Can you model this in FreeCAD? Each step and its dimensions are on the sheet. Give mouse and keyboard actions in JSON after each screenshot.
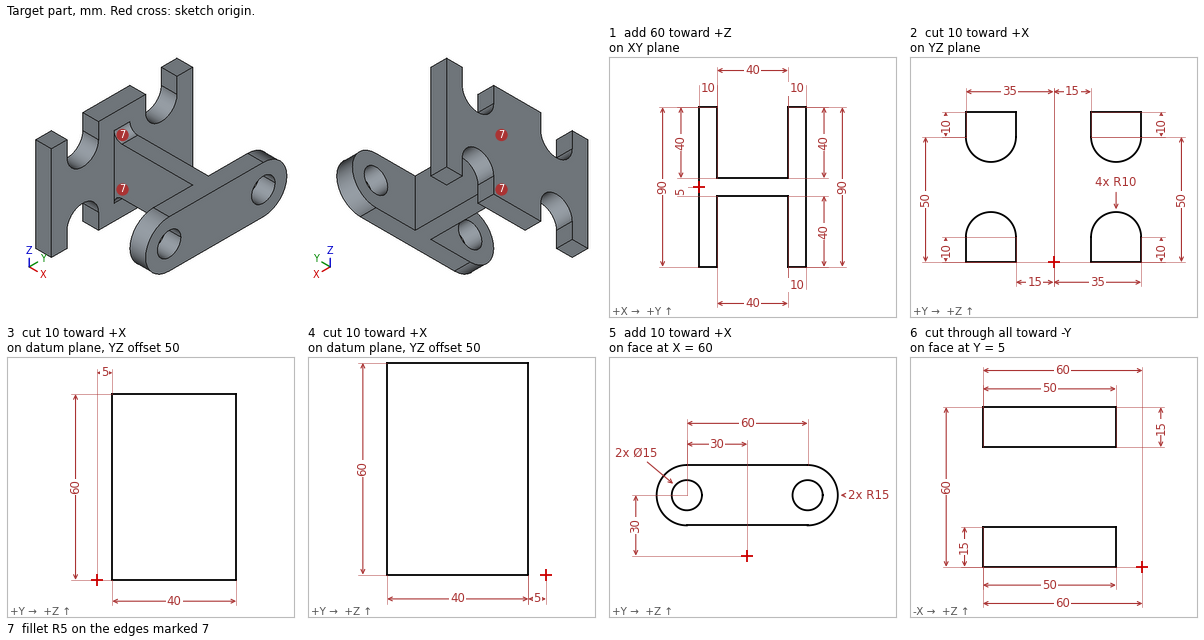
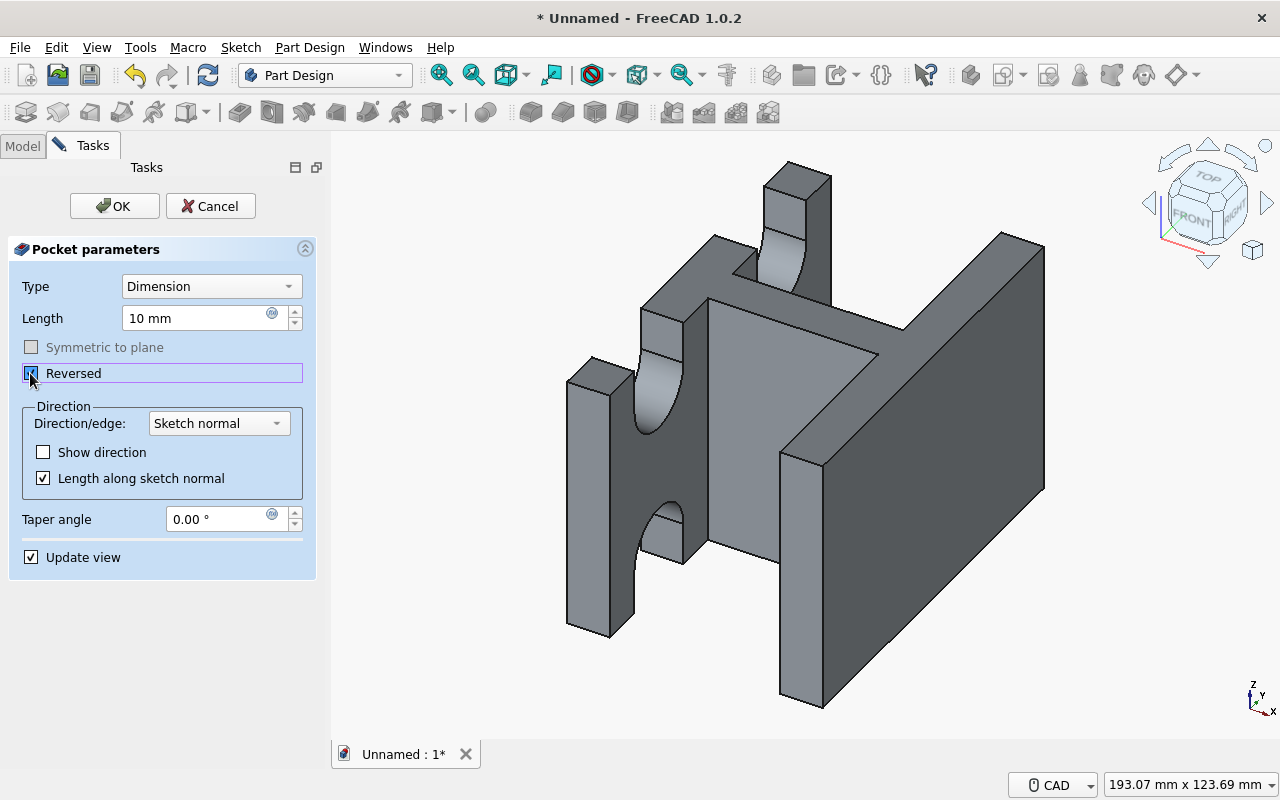
{"action": "left_click", "coordinate": [115, 206]}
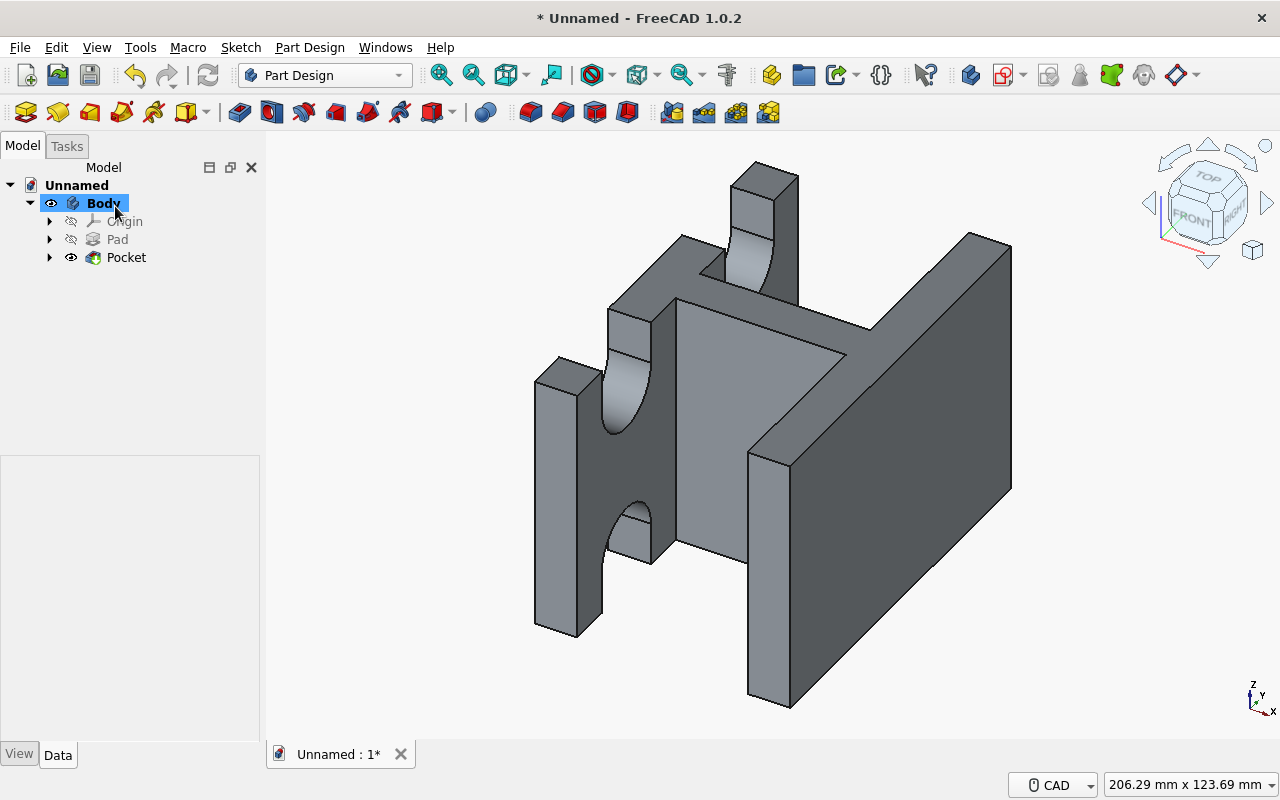
{"action": "left_click", "coordinate": [50, 221]}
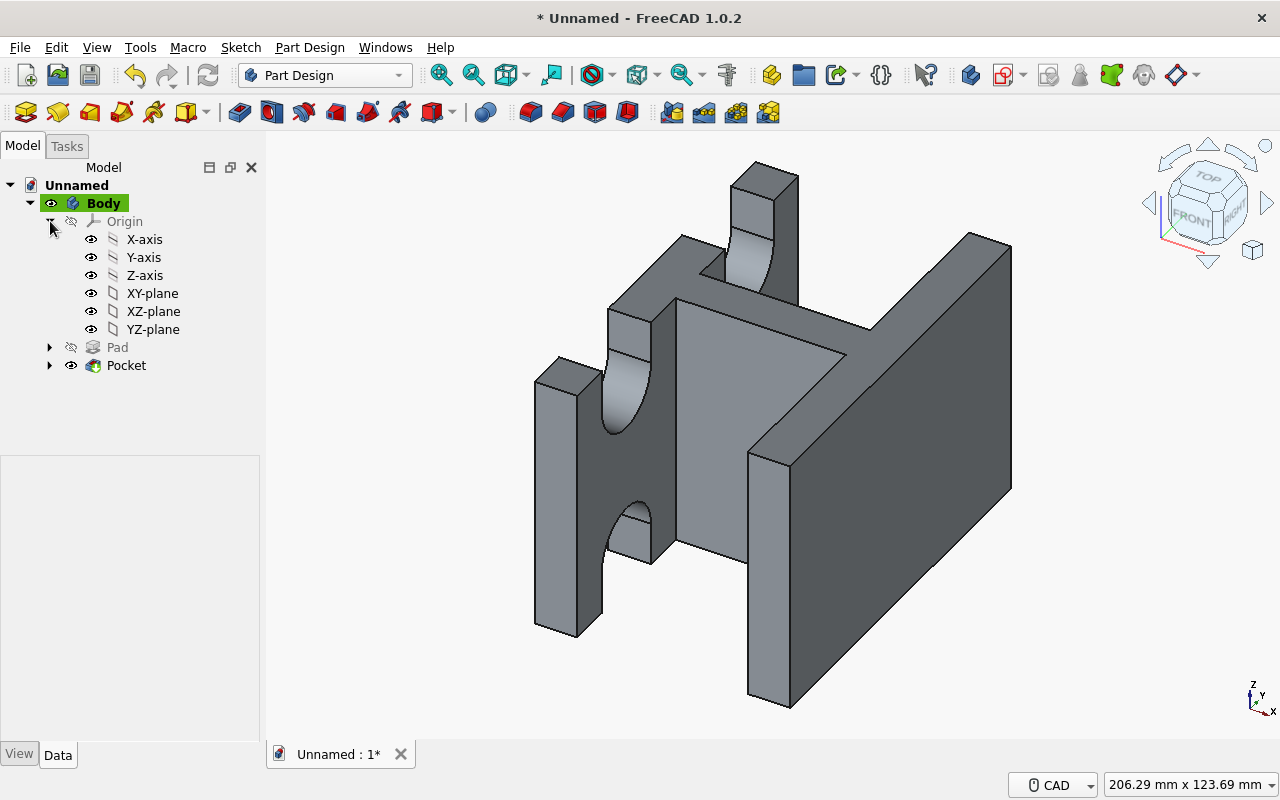
{"action": "left_click", "coordinate": [136, 329]}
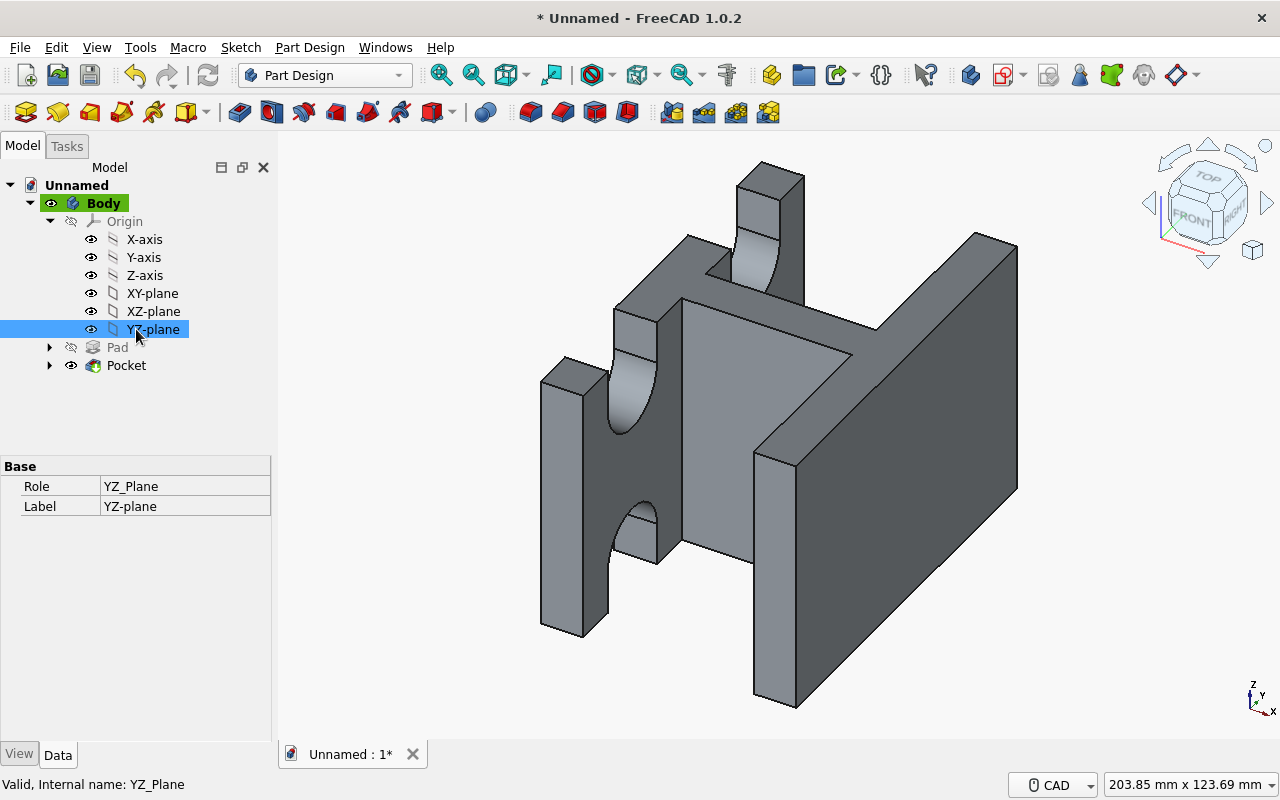
{"action": "left_click", "coordinate": [1176, 76]}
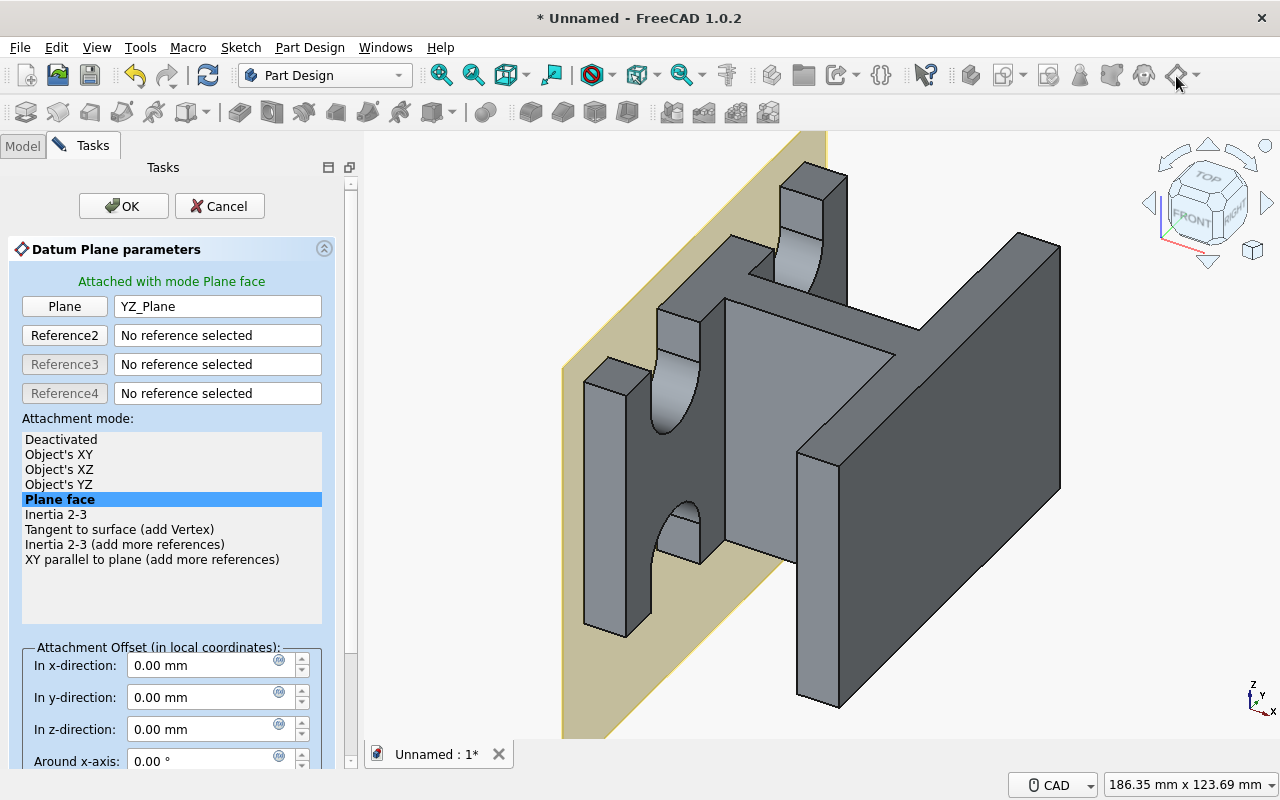
{"action": "triple_click", "coordinate": [210, 729]}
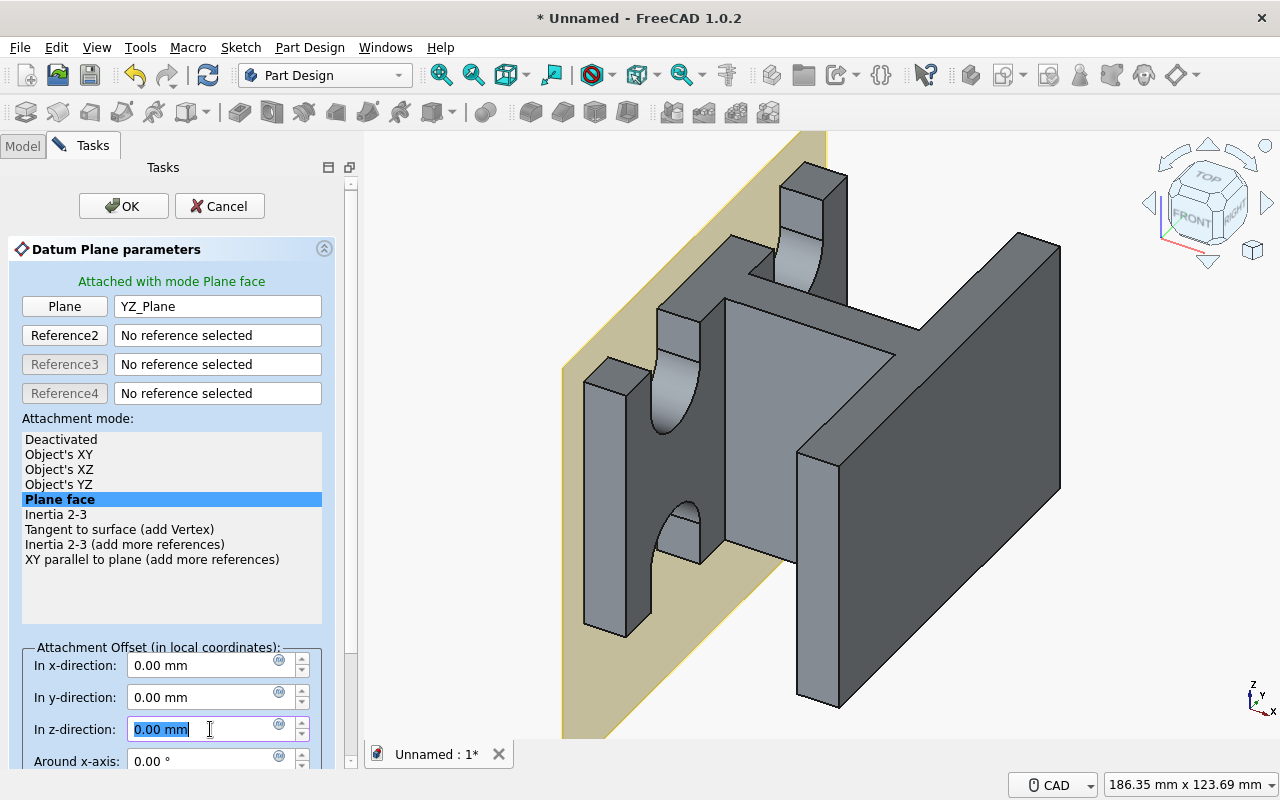
{"action": "type", "text": "50"}
{"action": "key", "text": "Tab"}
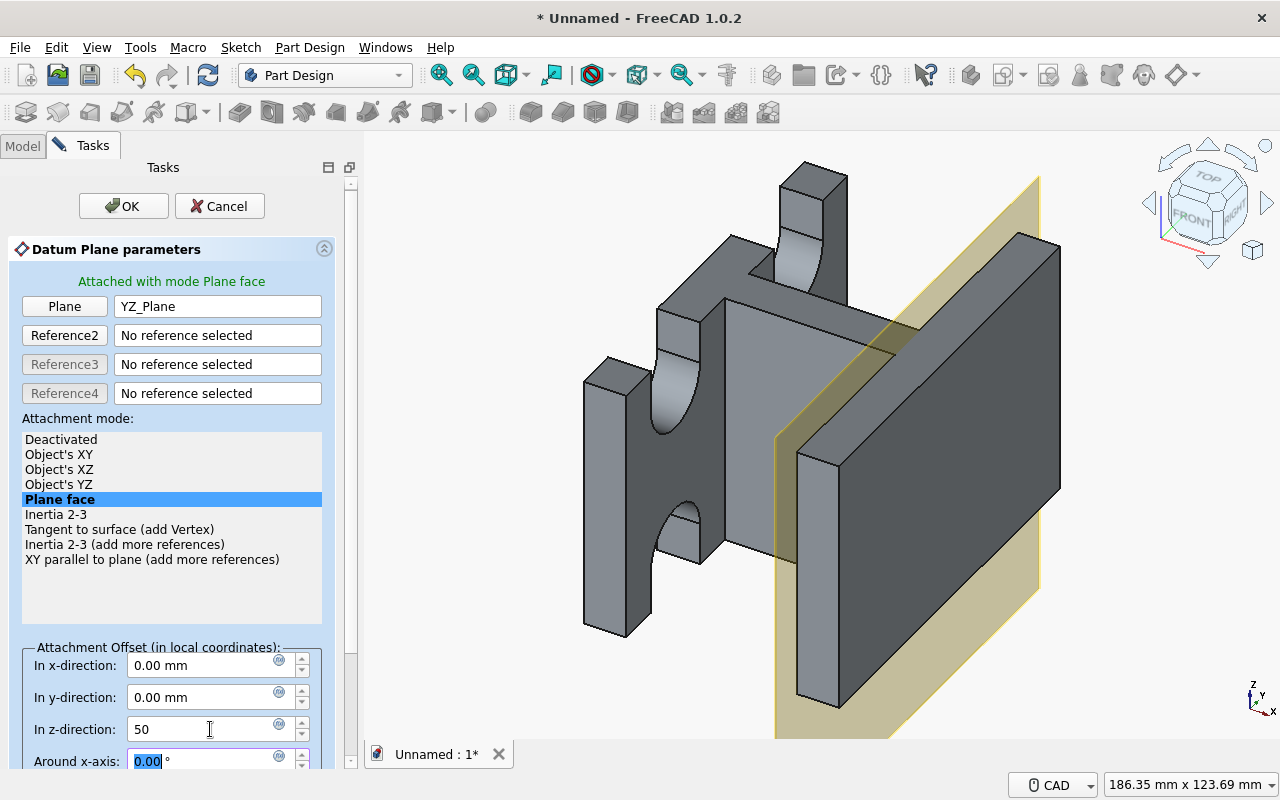
{"action": "left_click", "coordinate": [124, 206]}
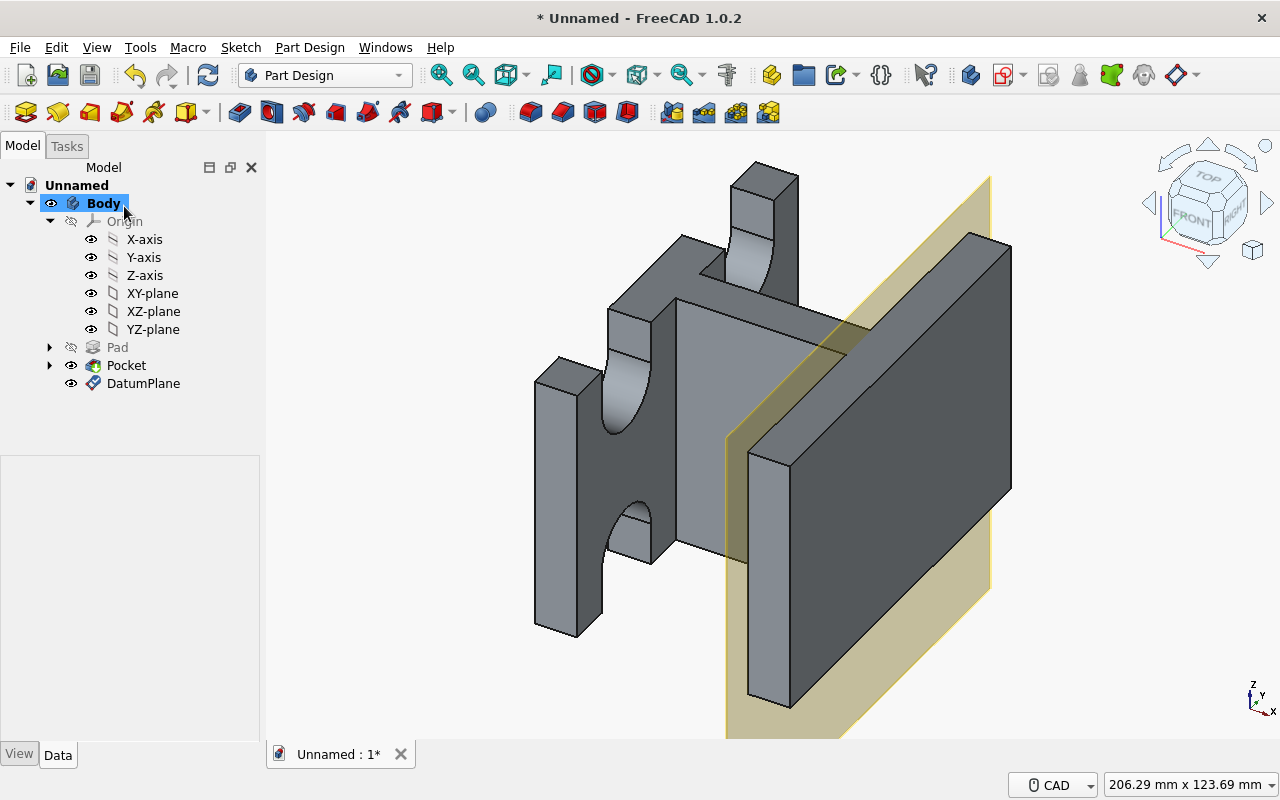
{"action": "left_click", "coordinate": [116, 383]}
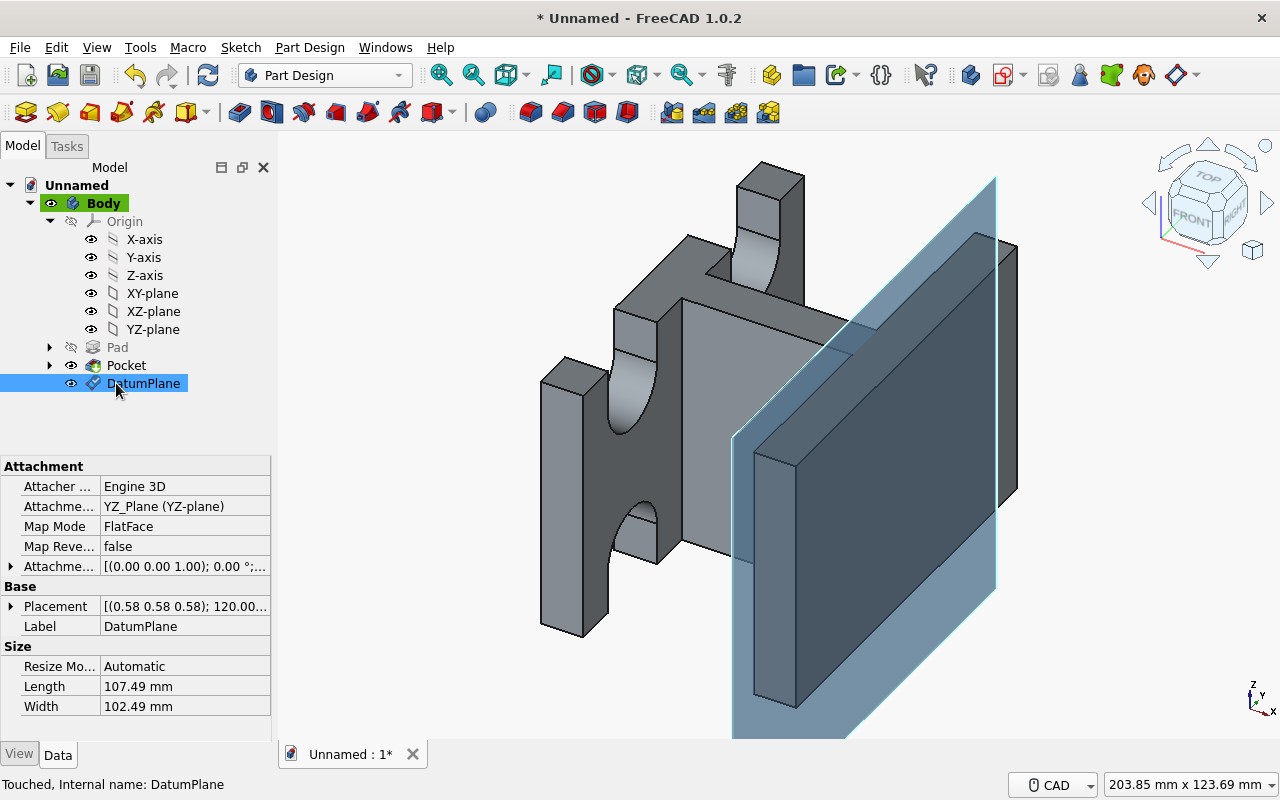
{"action": "left_click", "coordinate": [1004, 76]}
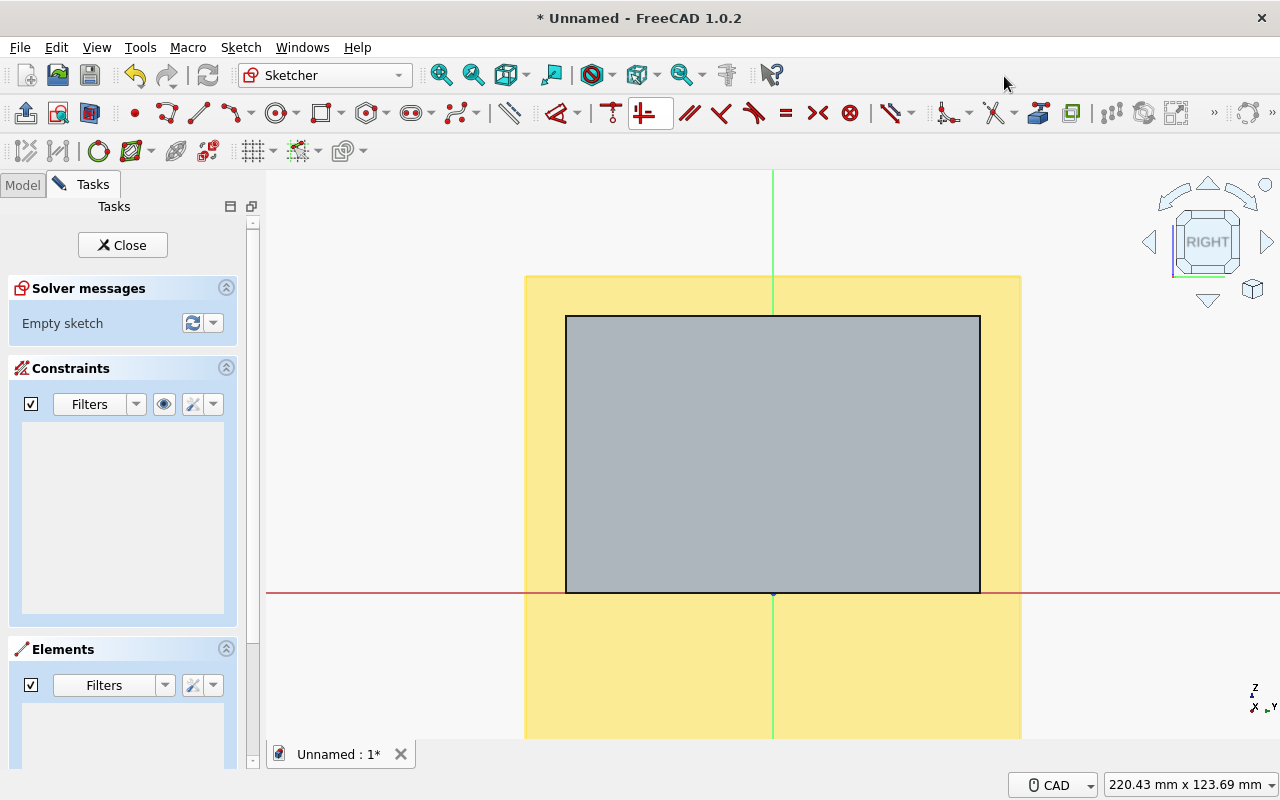
{"action": "left_click", "coordinate": [90, 114]}